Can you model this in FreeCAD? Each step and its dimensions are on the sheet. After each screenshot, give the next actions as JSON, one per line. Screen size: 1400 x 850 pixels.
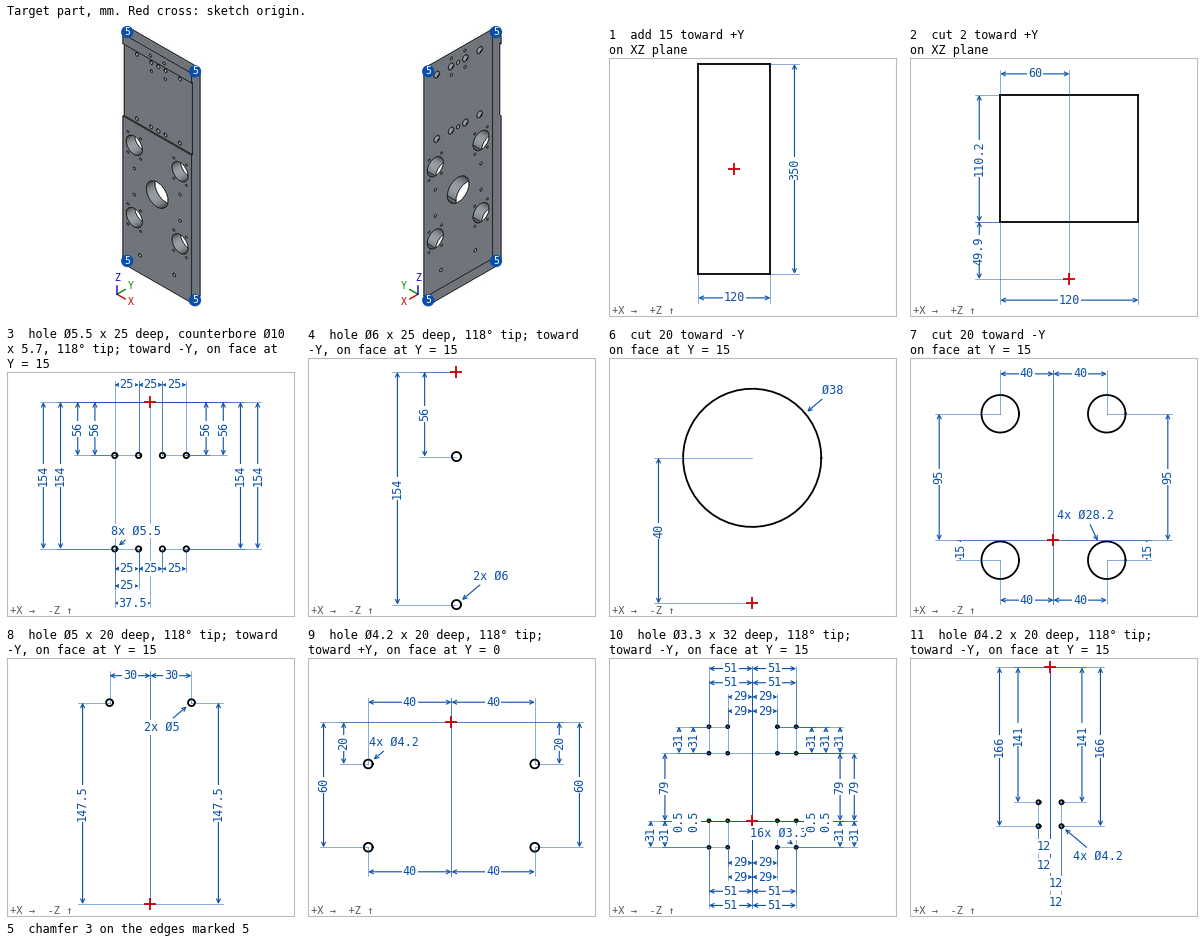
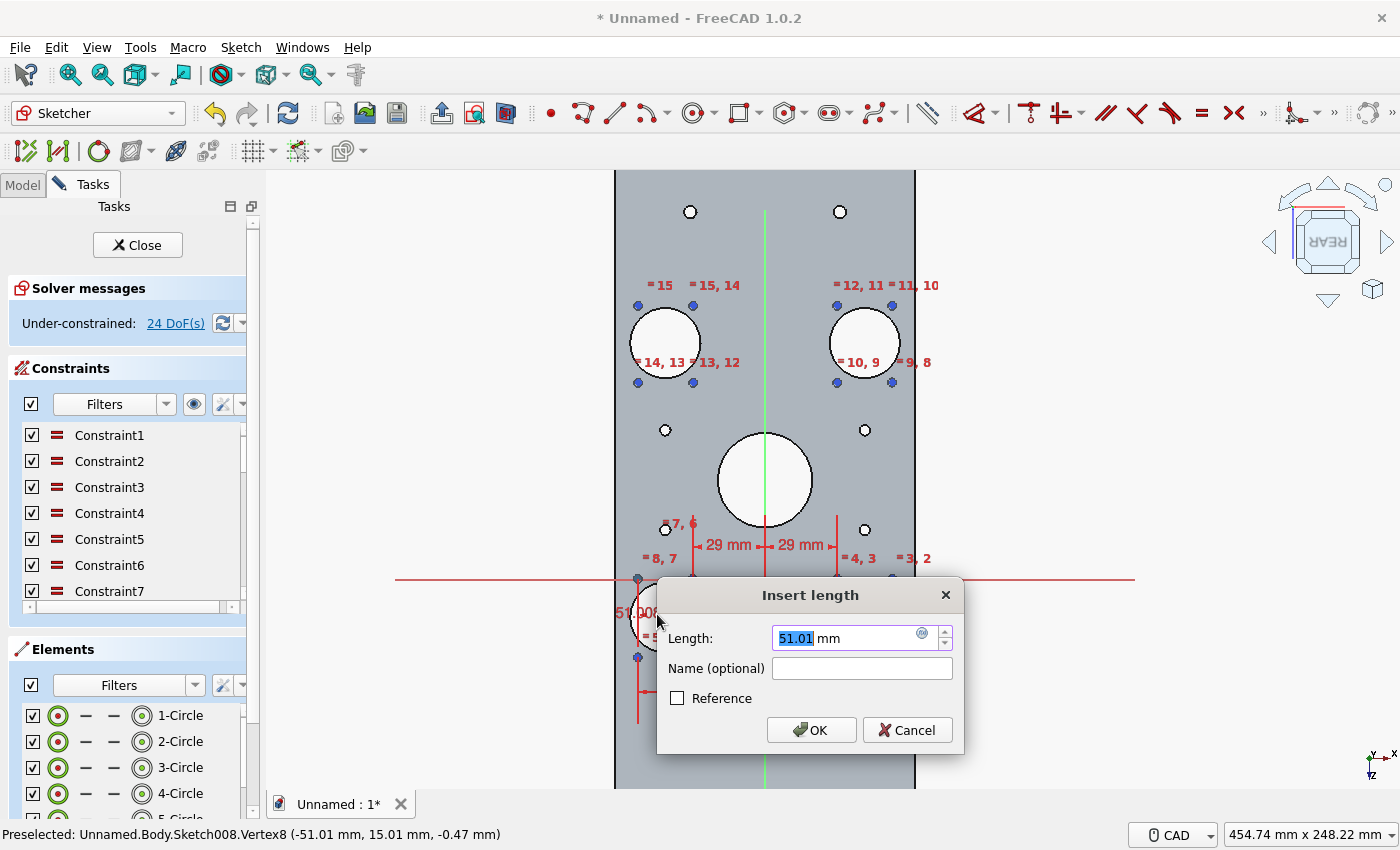
{"action": "type", "text": "51"}
{"action": "key", "text": "Return"}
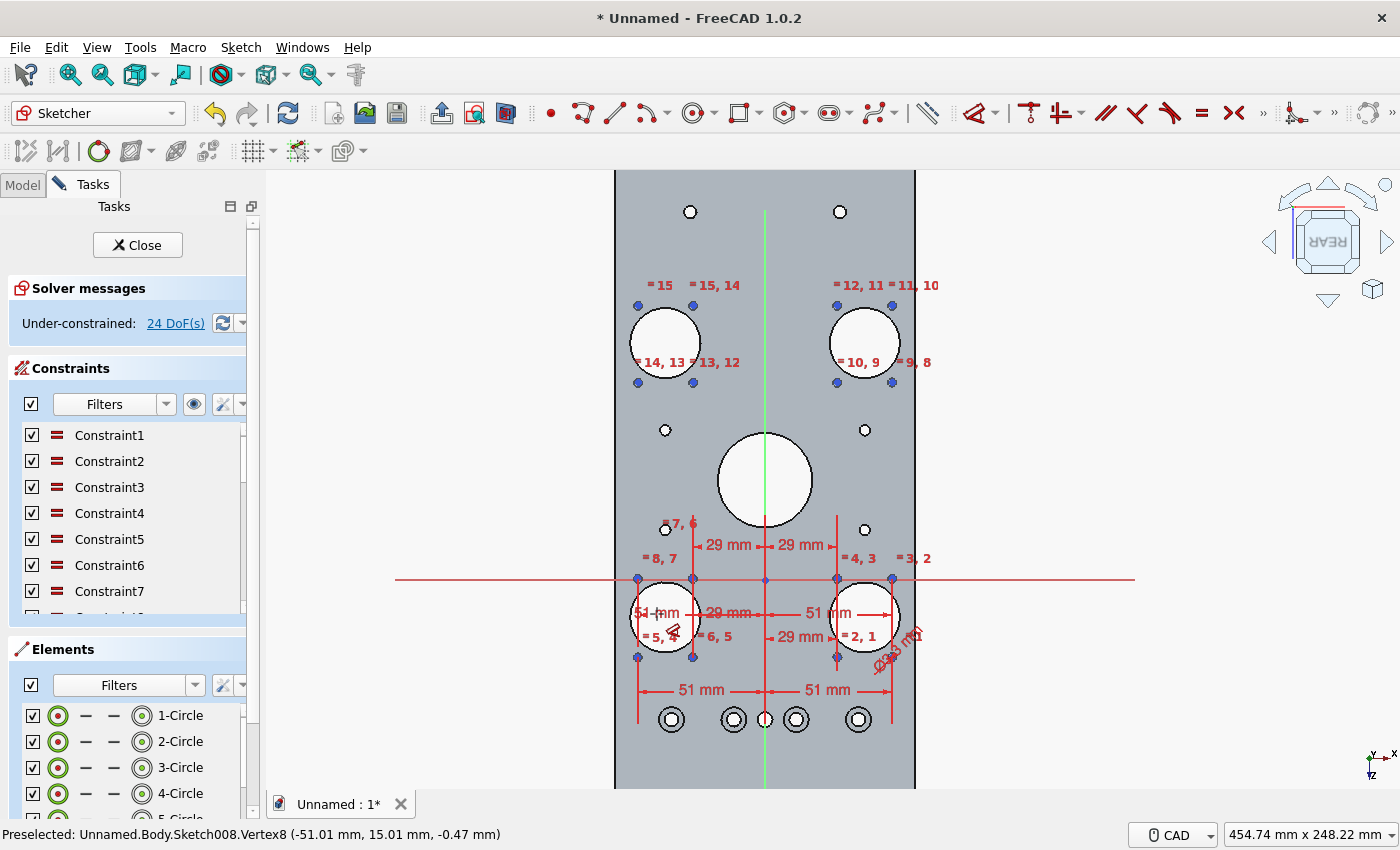
{"action": "left_click", "coordinate": [892, 383]}
{"action": "left_click", "coordinate": [829, 349]}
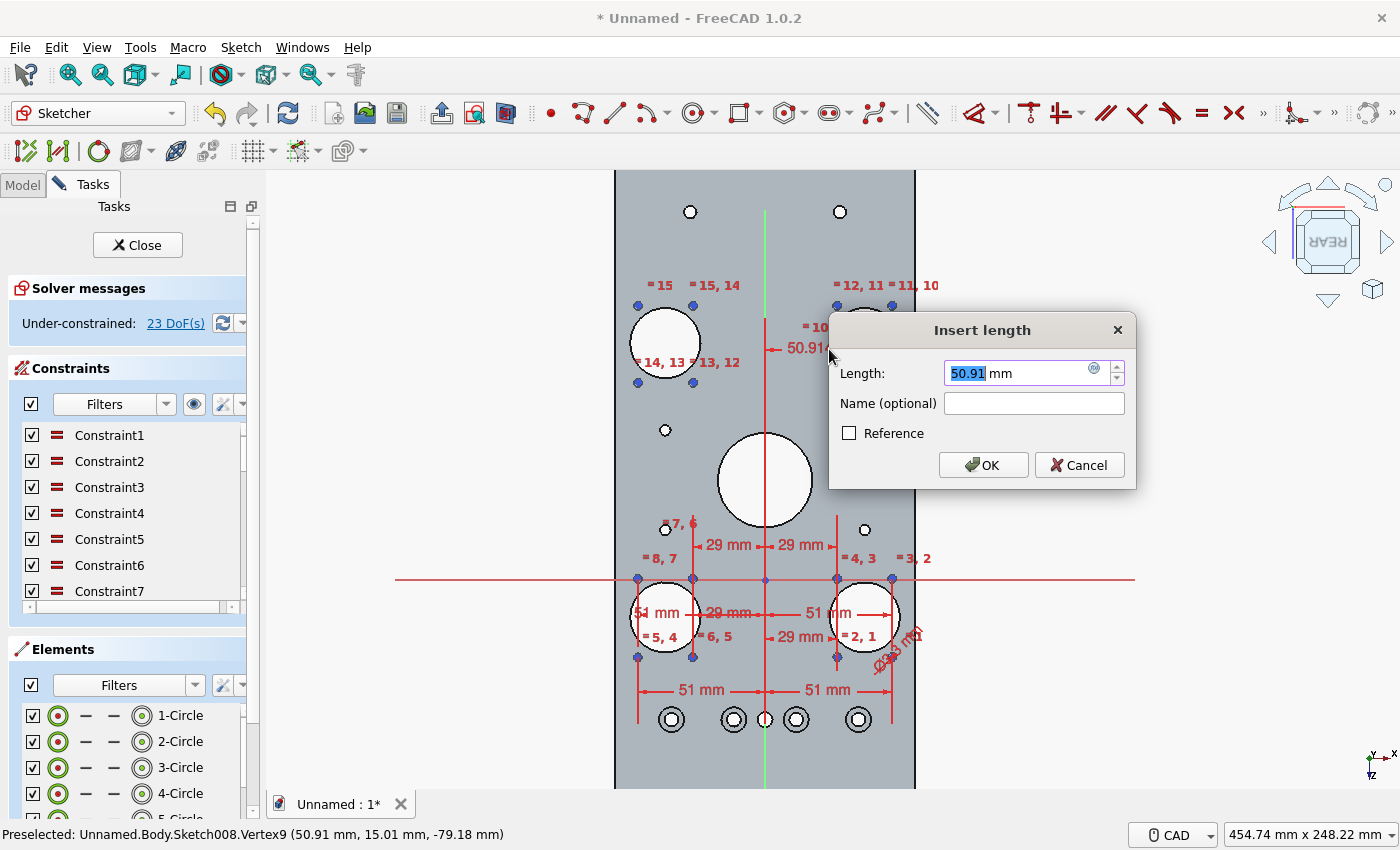
{"action": "type", "text": "51"}
{"action": "key", "text": "Return"}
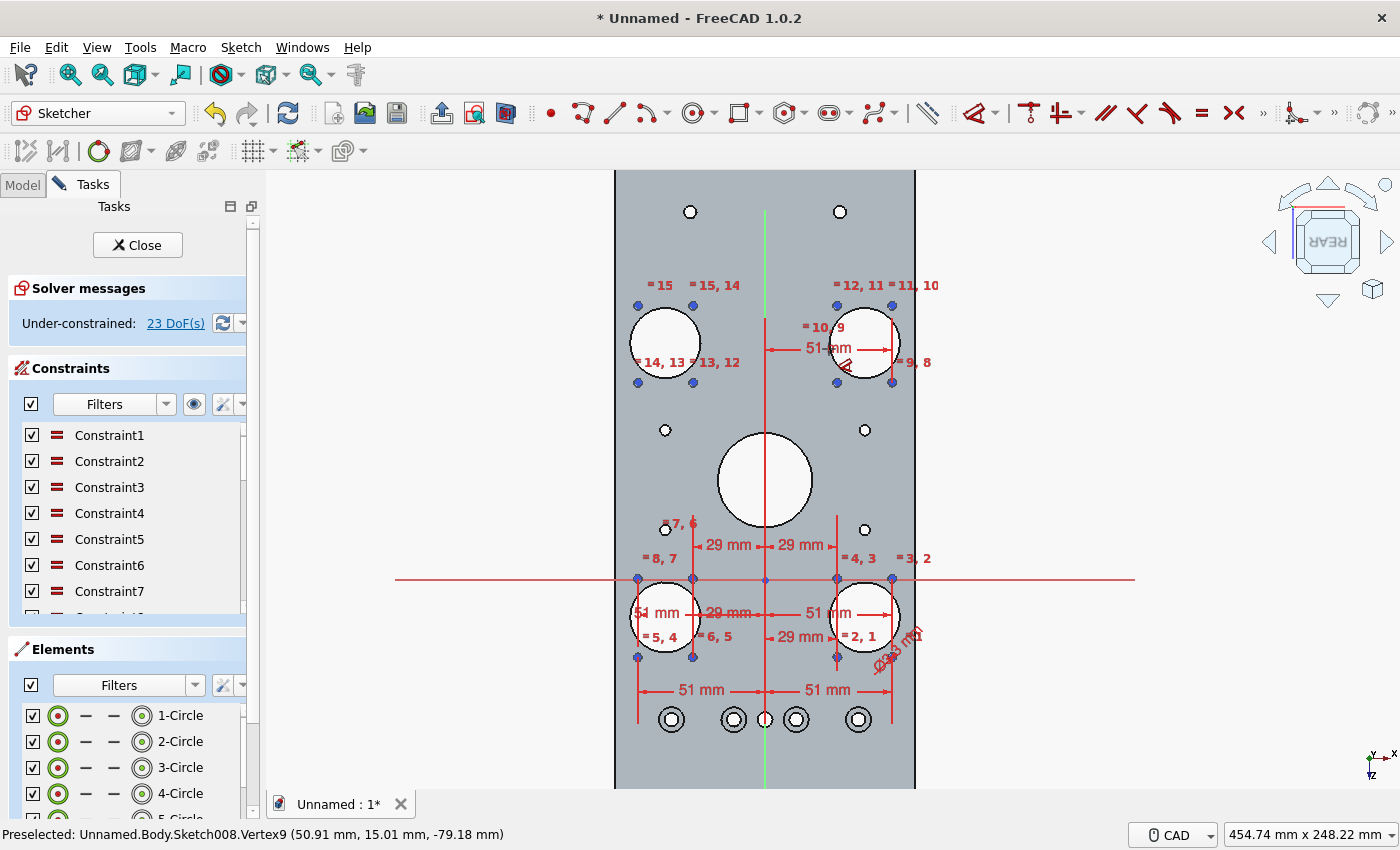
{"action": "left_click", "coordinate": [837, 383]}
{"action": "left_click", "coordinate": [801, 325]}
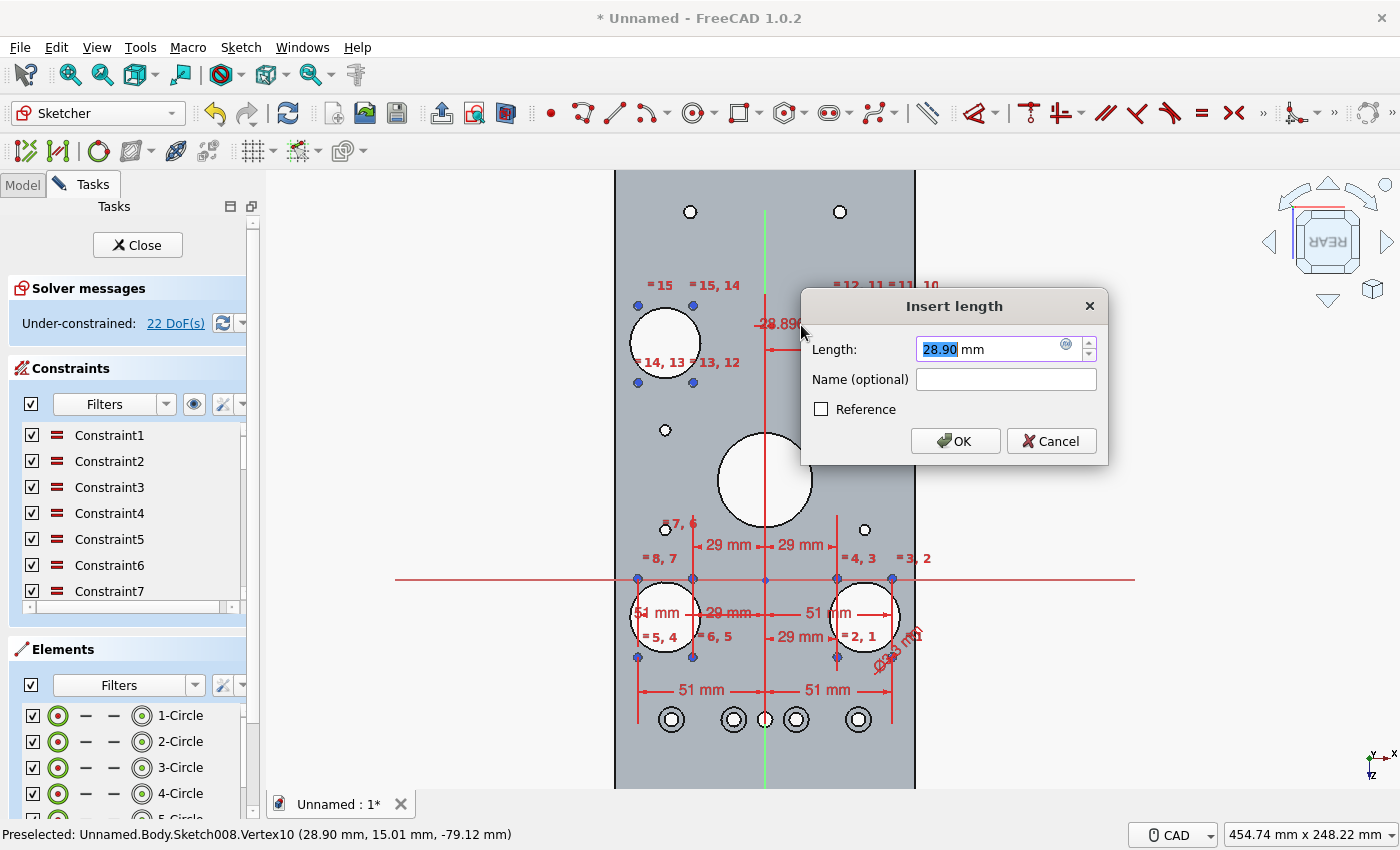
{"action": "type", "text": "29"}
{"action": "key", "text": "Return"}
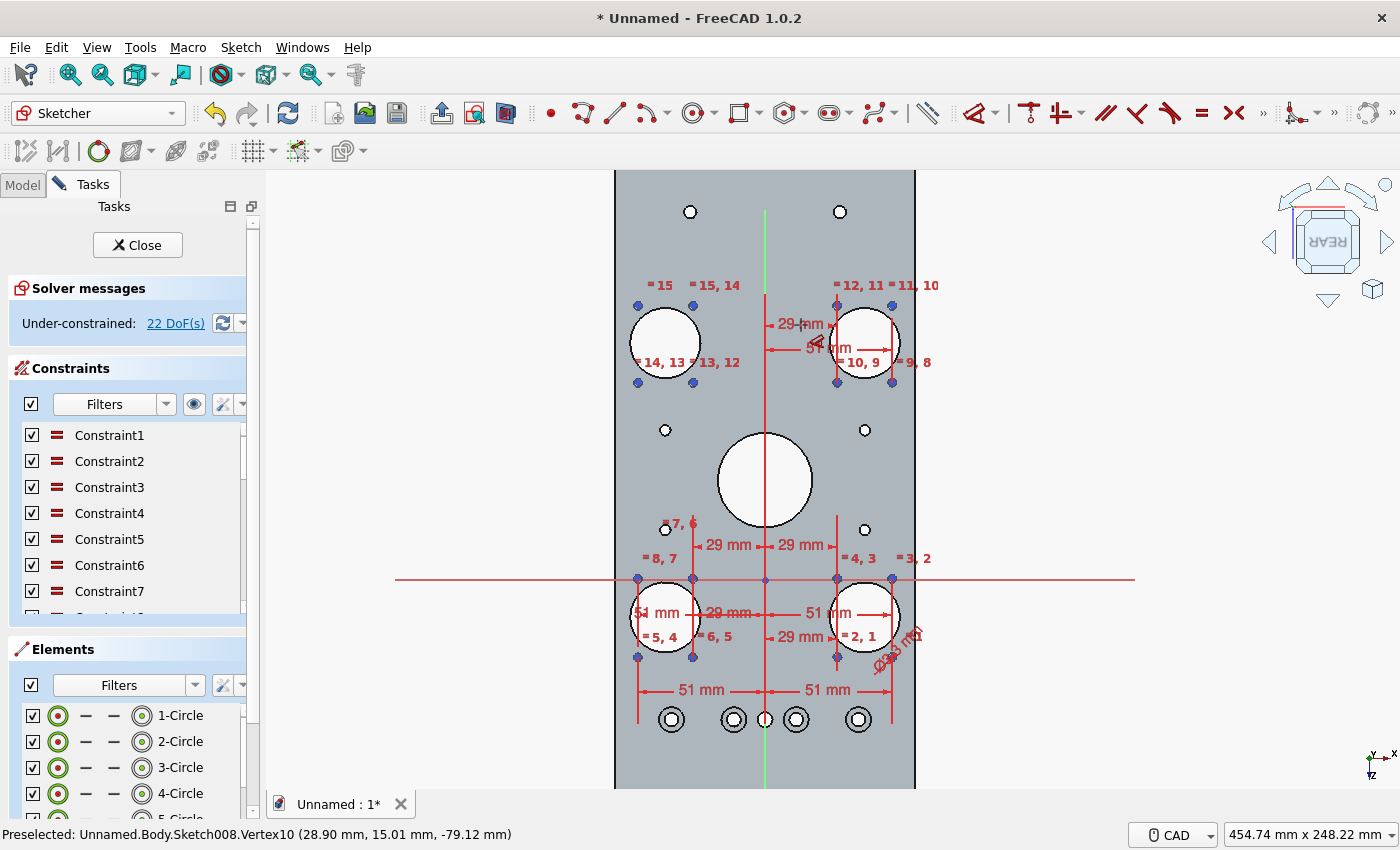
{"action": "left_click", "coordinate": [892, 306]}
{"action": "left_click", "coordinate": [829, 272]}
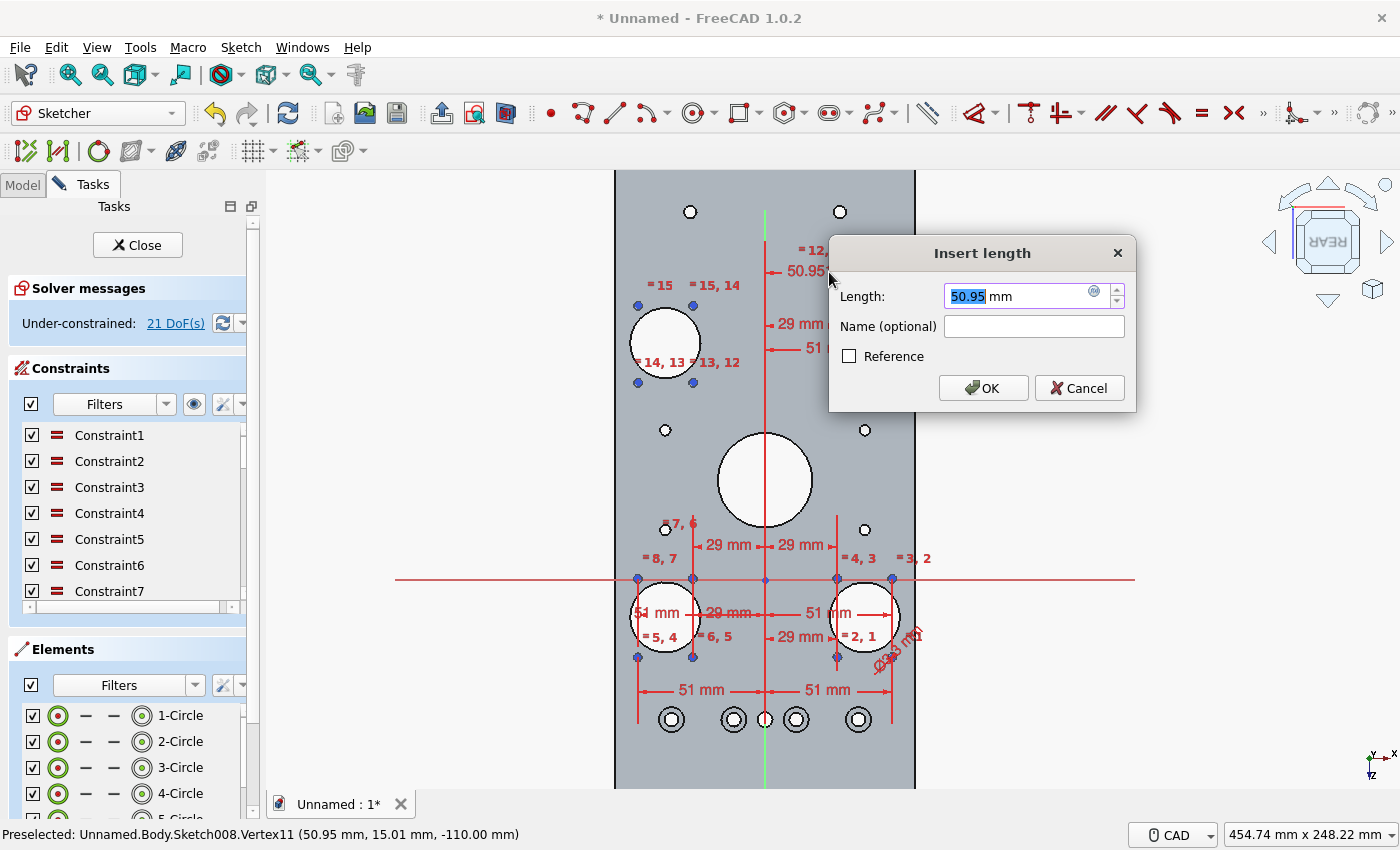
{"action": "type", "text": "51"}
{"action": "key", "text": "Return"}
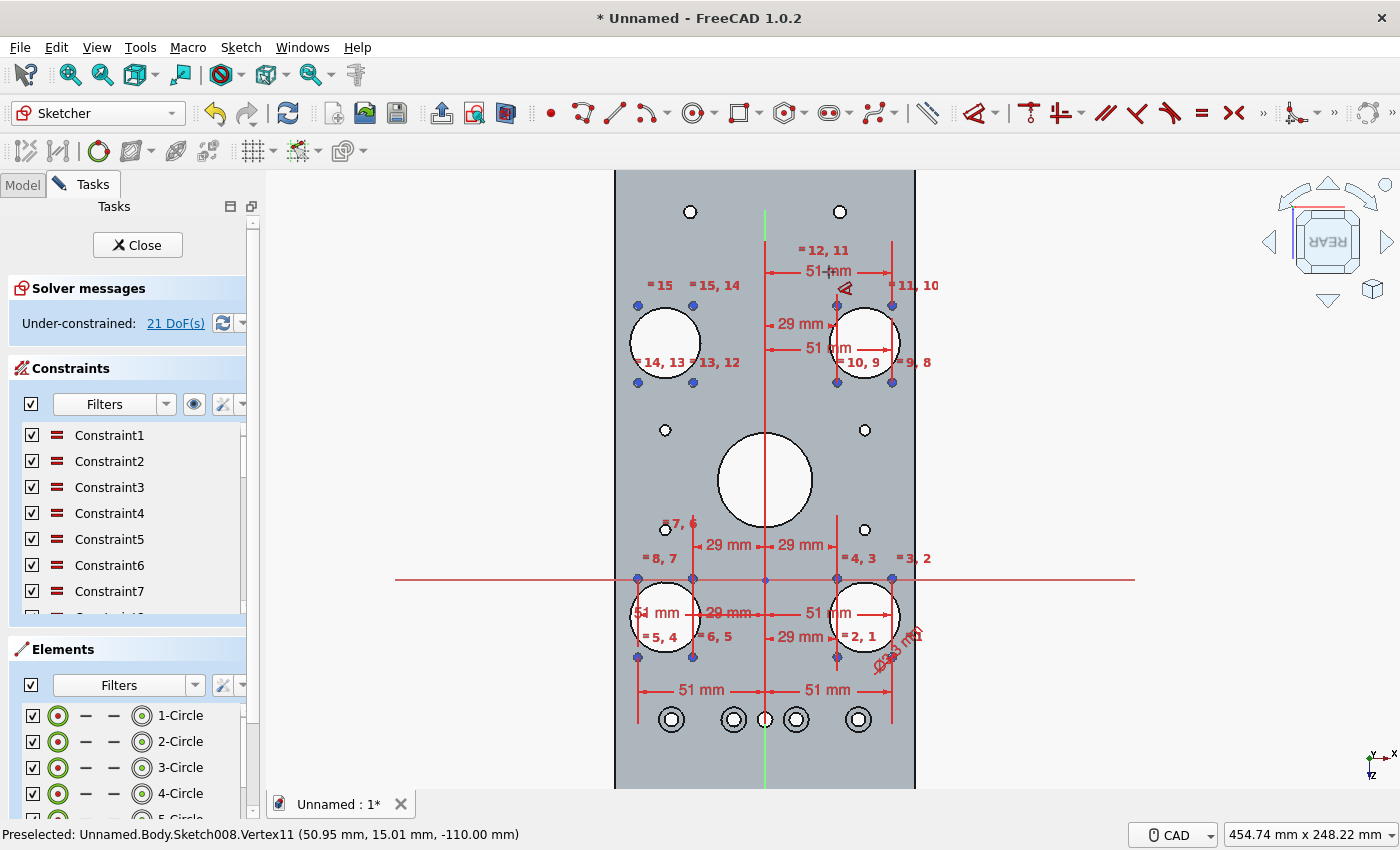
{"action": "left_click", "coordinate": [837, 306]}
{"action": "left_click", "coordinate": [801, 248]}